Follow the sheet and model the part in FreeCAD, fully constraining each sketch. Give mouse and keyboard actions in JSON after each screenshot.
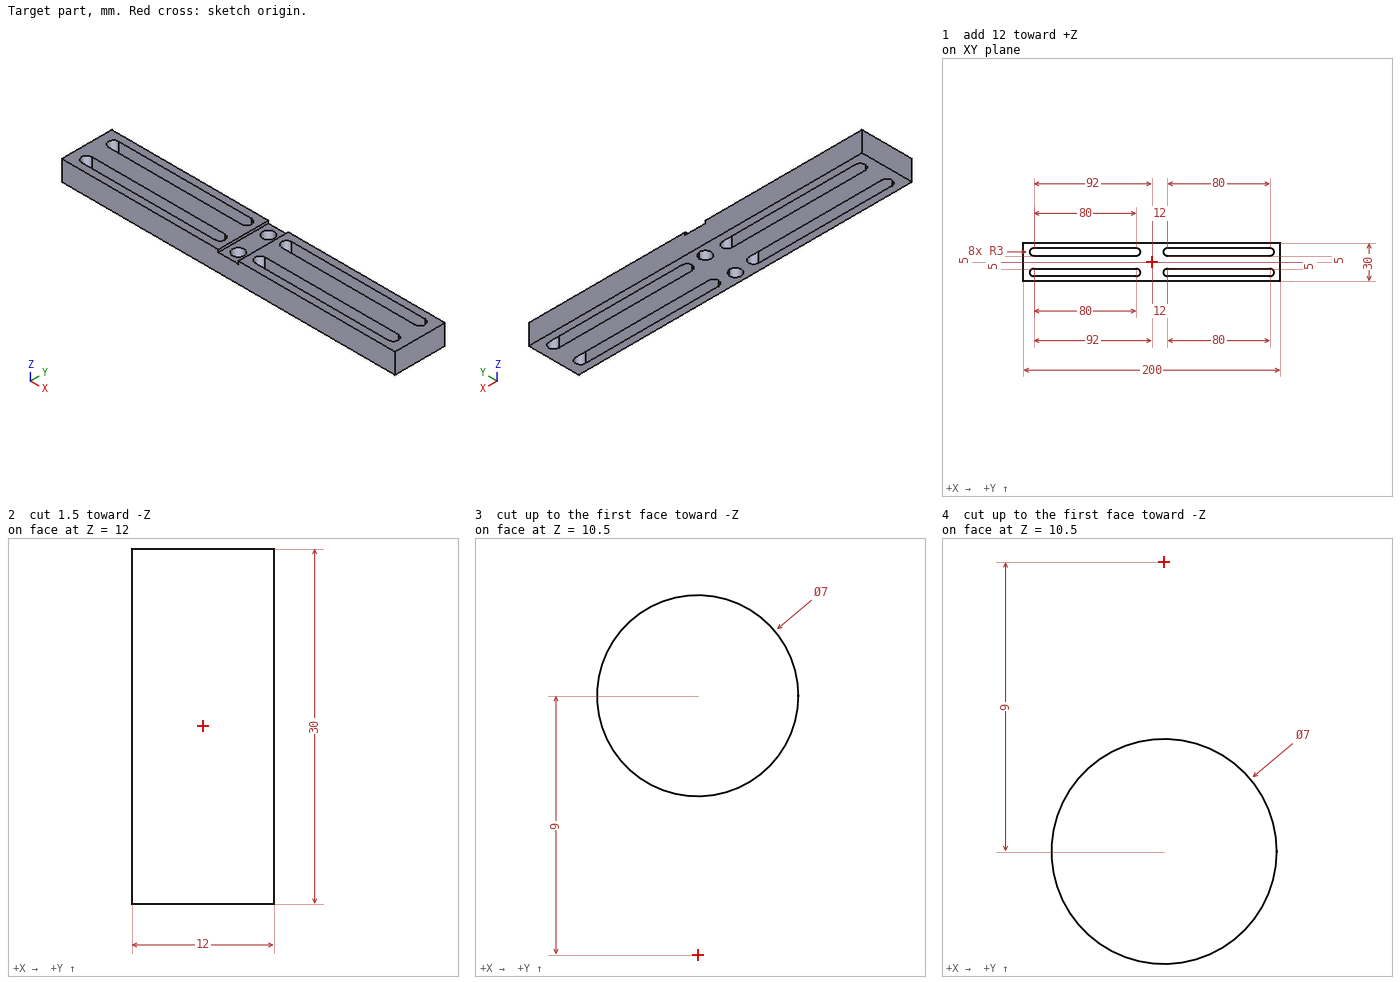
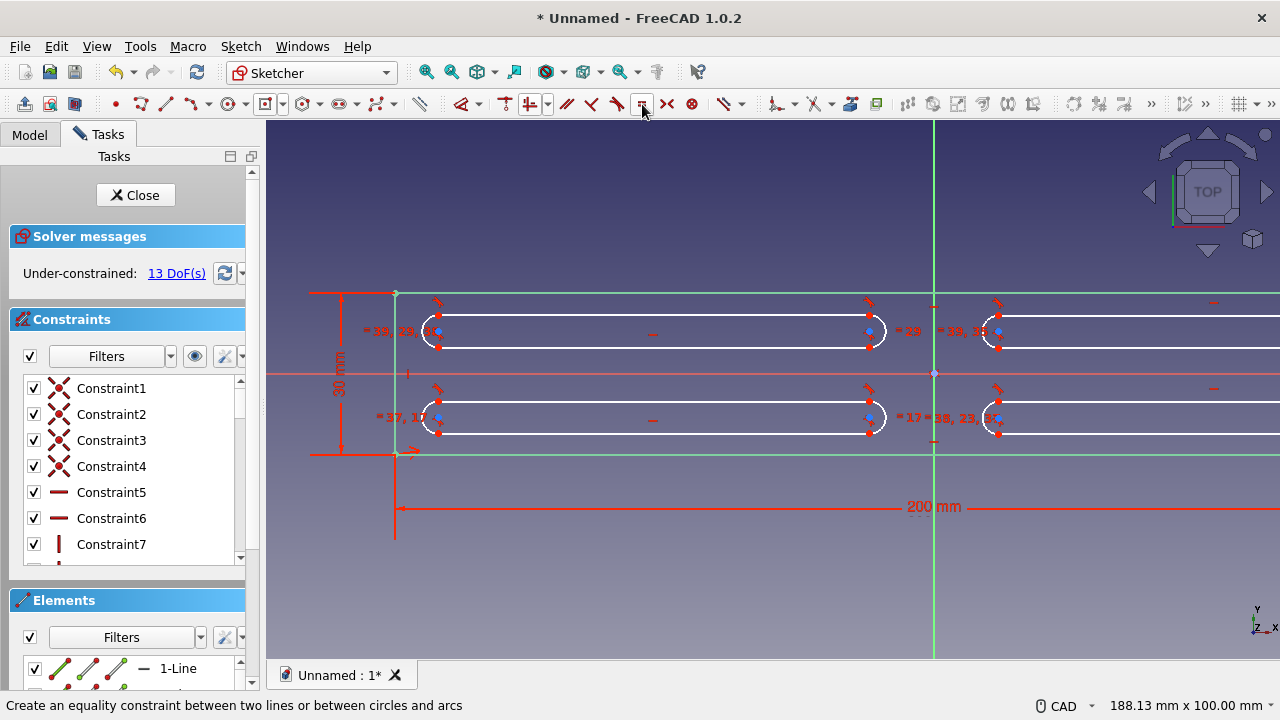
{"action": "left_click", "coordinate": [460, 104]}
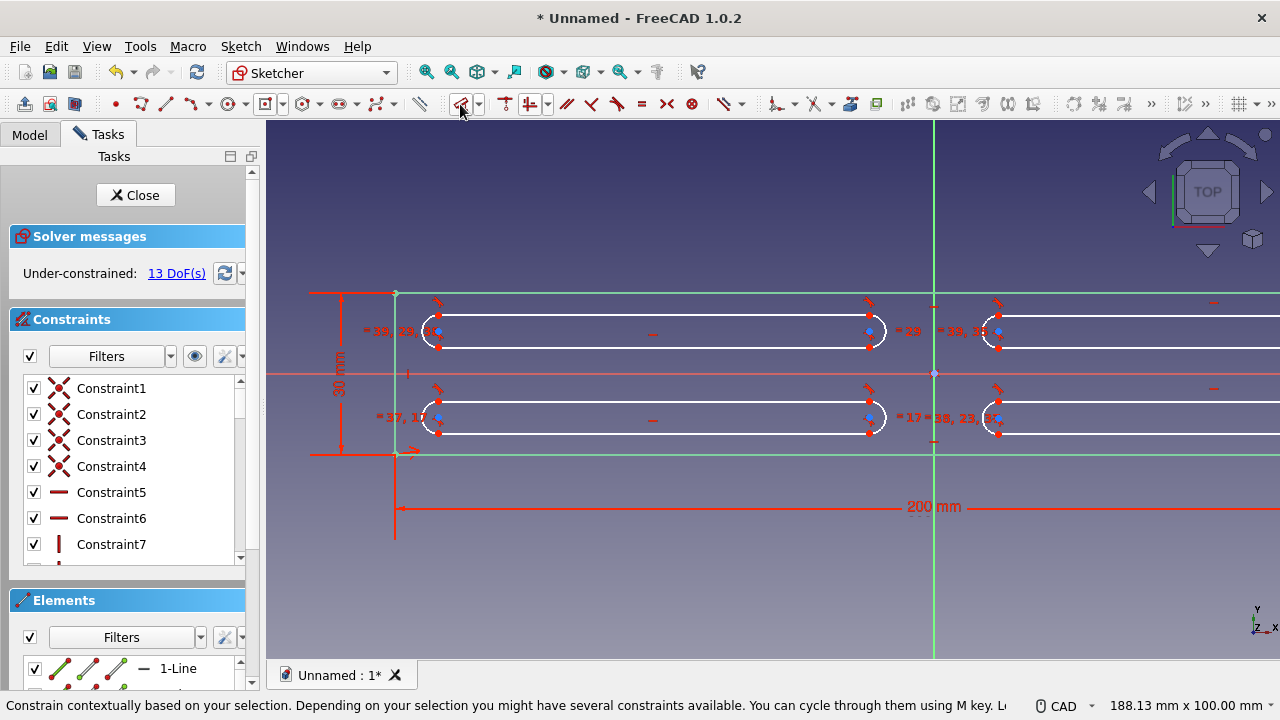
{"action": "scroll", "coordinate": [425, 408], "scroll_direction": "up", "scroll_amount": 5}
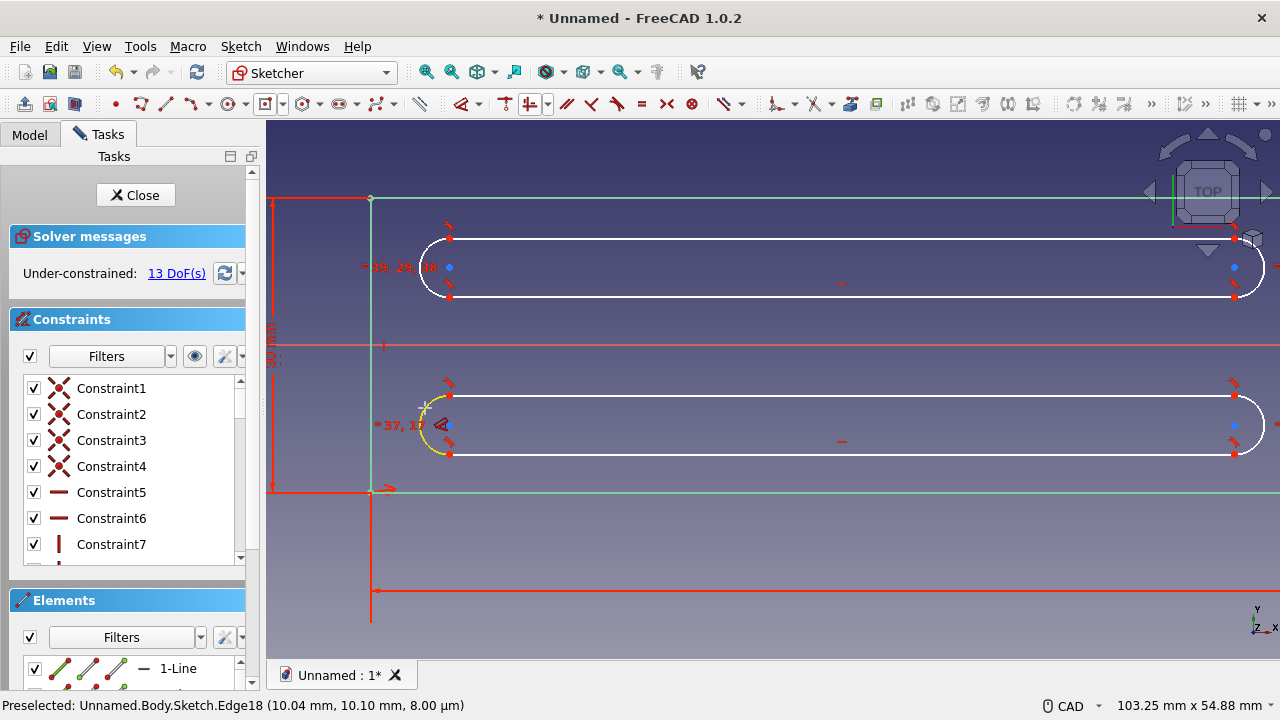
{"action": "left_click", "coordinate": [426, 408]}
{"action": "left_click", "coordinate": [400, 389]}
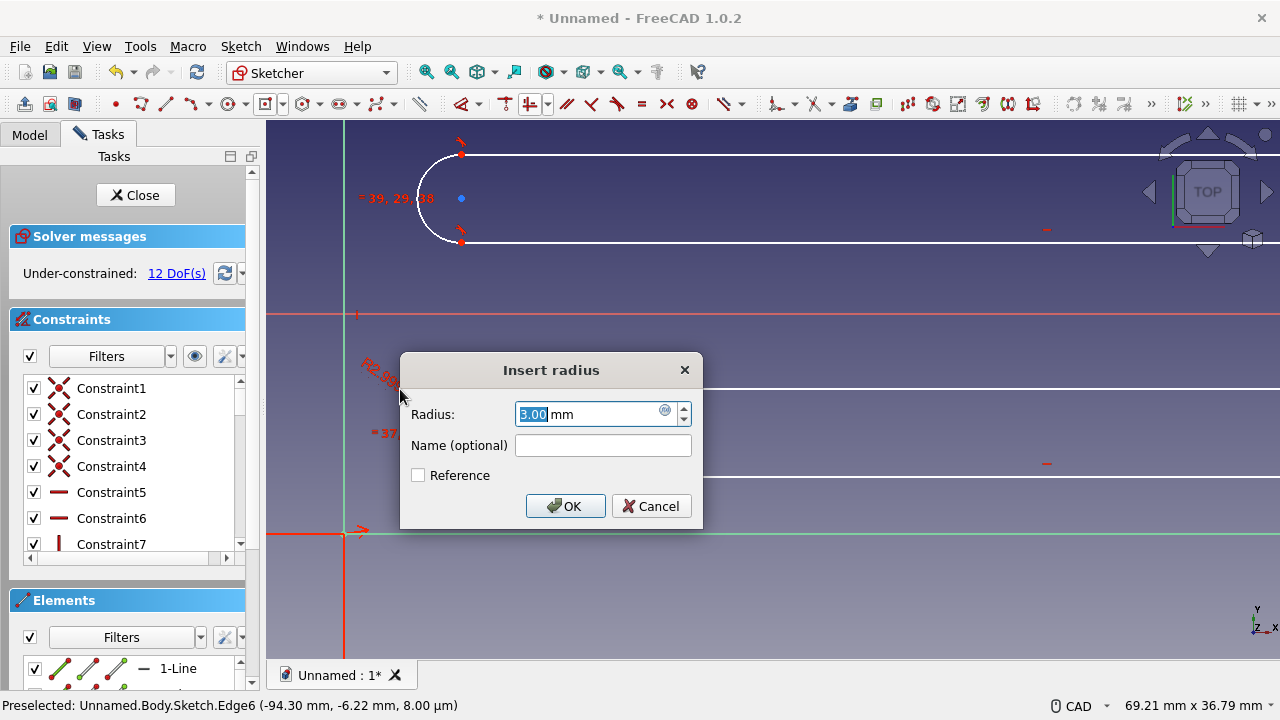
{"action": "type", "text": "3"}
{"action": "key", "text": "Return"}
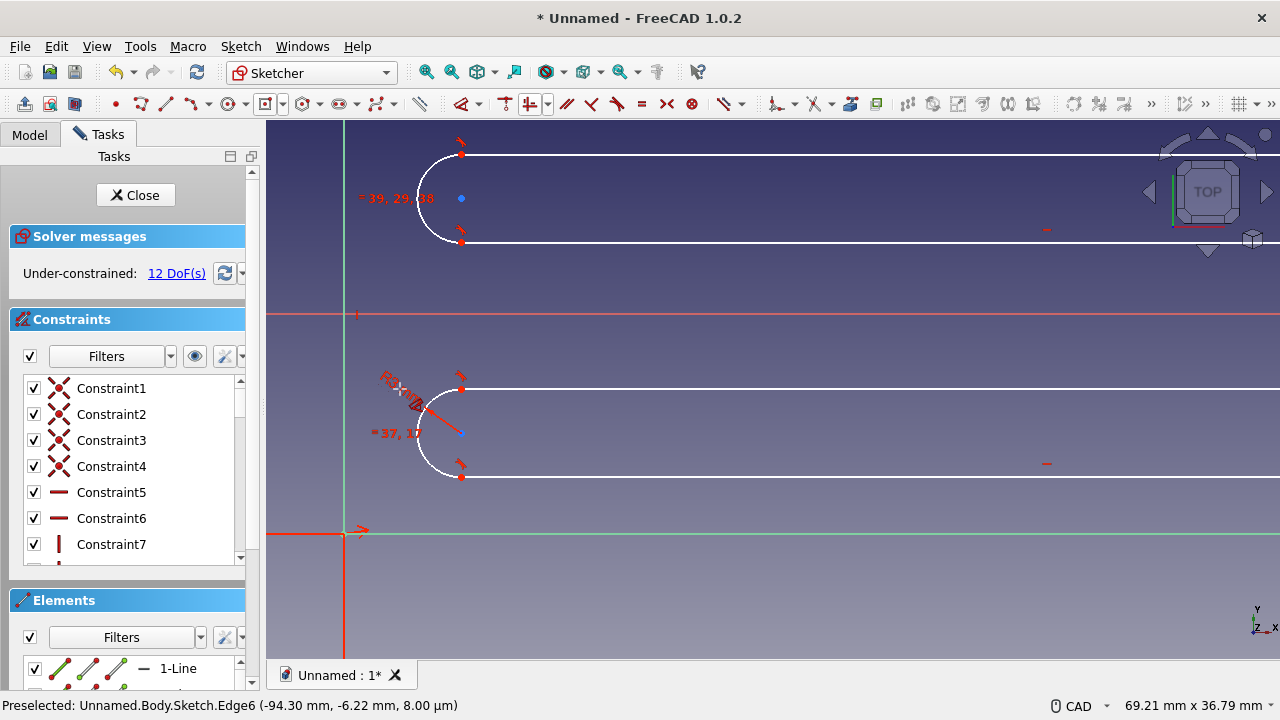
{"action": "scroll", "coordinate": [425, 409], "scroll_direction": "down", "scroll_amount": 8}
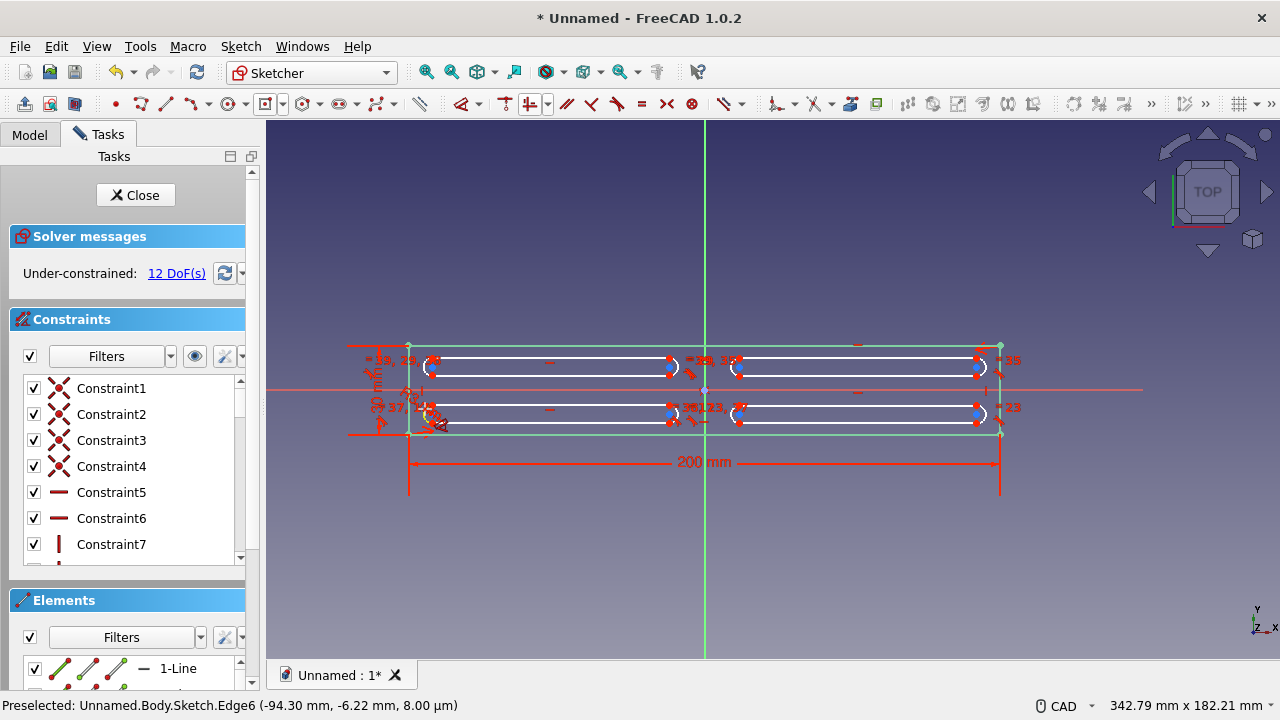
{"action": "left_click", "coordinate": [503, 405]}
{"action": "left_click", "coordinate": [551, 463]}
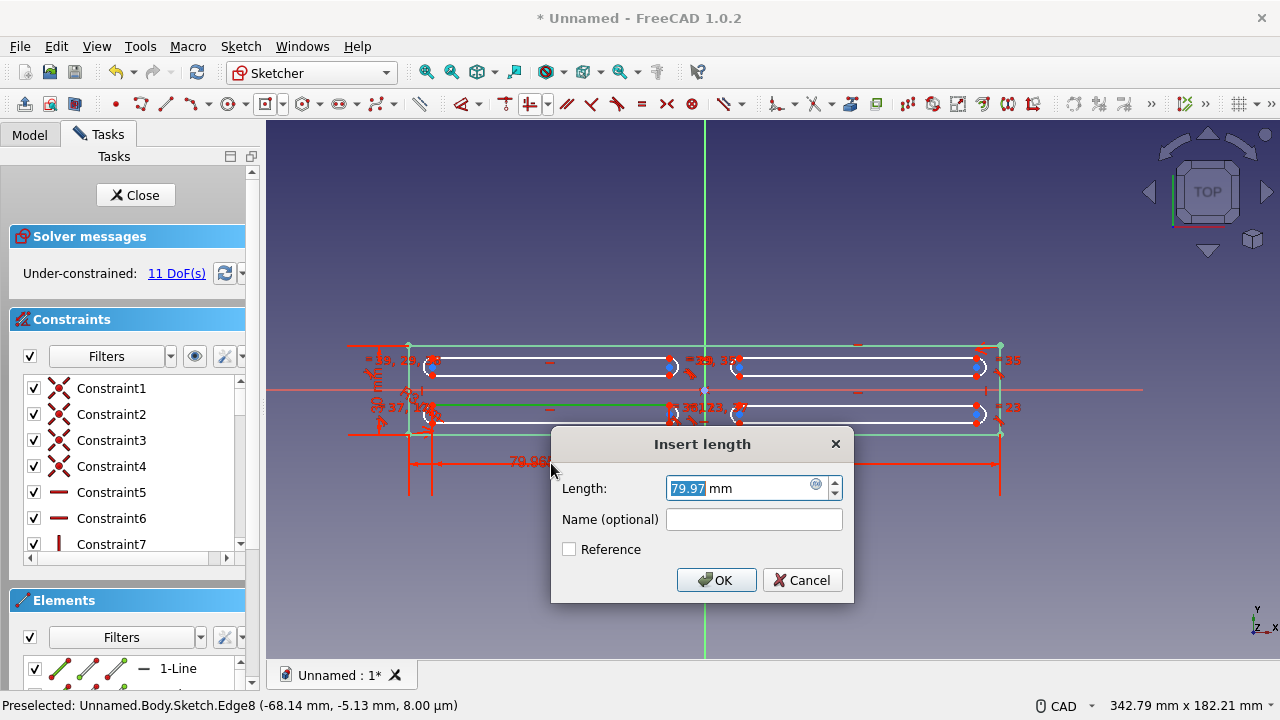
{"action": "type", "text": "80"}
{"action": "key", "text": "Return"}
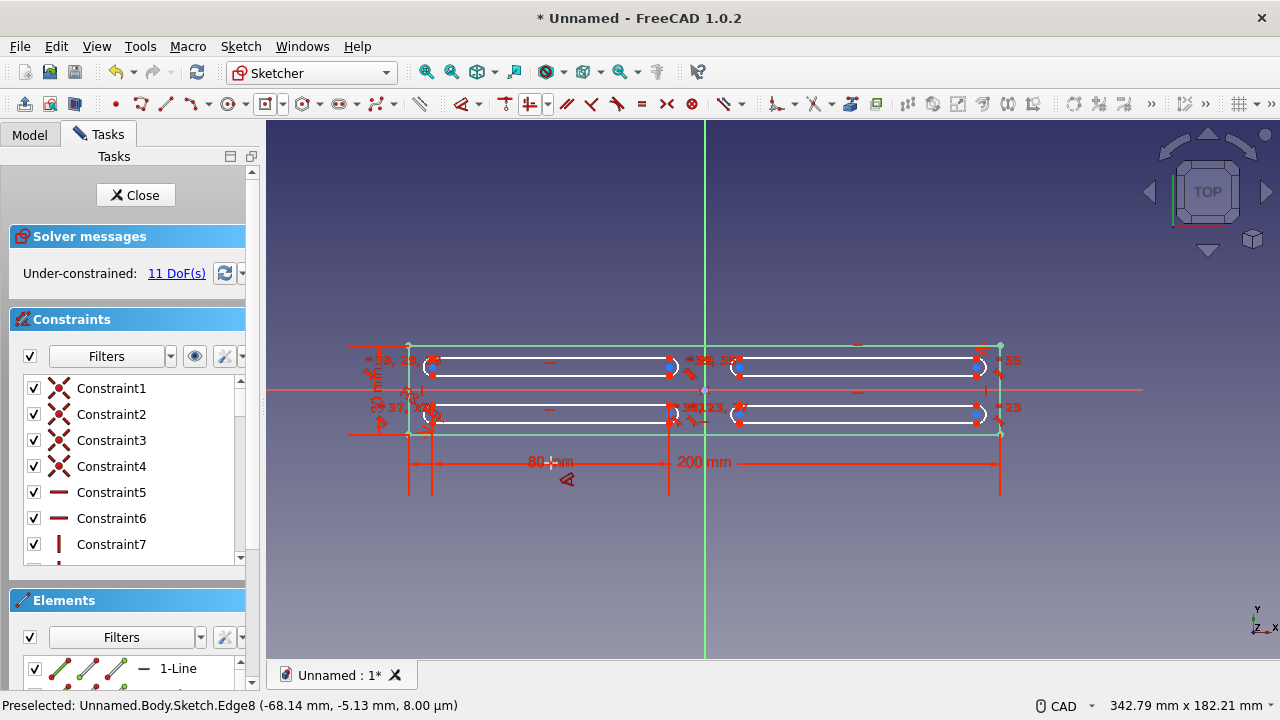
{"action": "left_click", "coordinate": [811, 406]}
{"action": "left_click", "coordinate": [858, 464]}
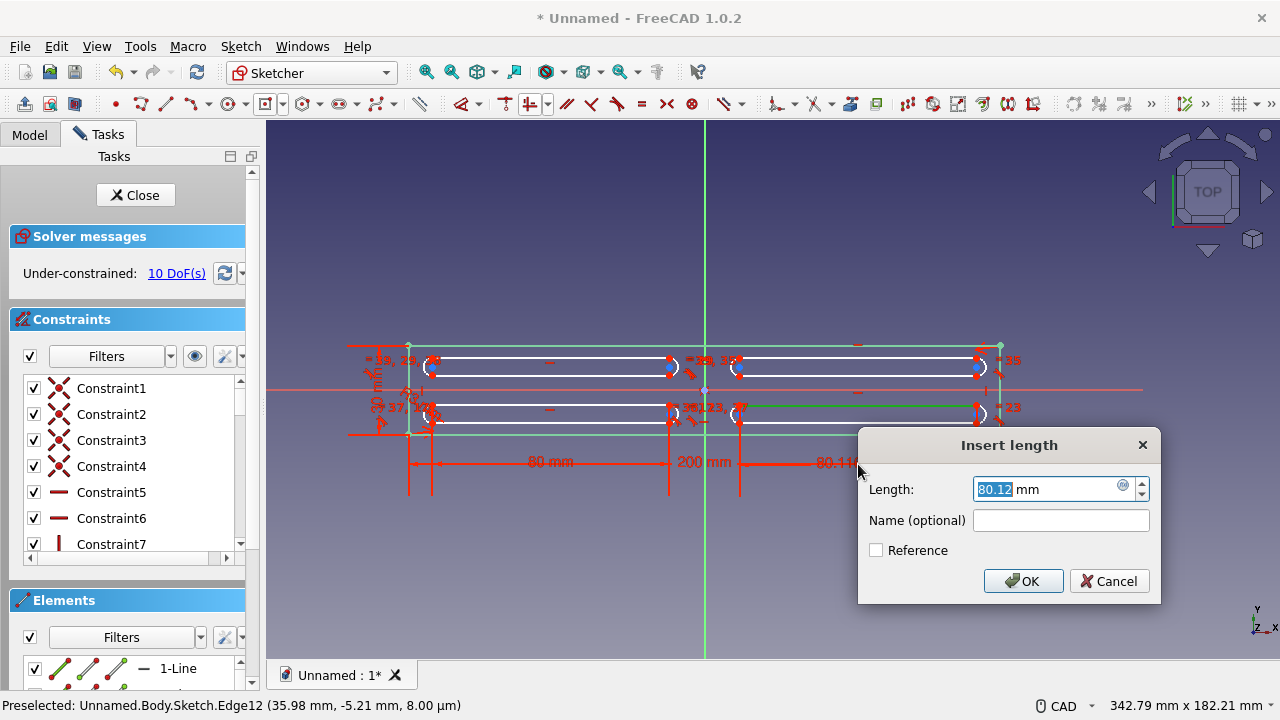
{"action": "type", "text": "80"}
{"action": "key", "text": "Return"}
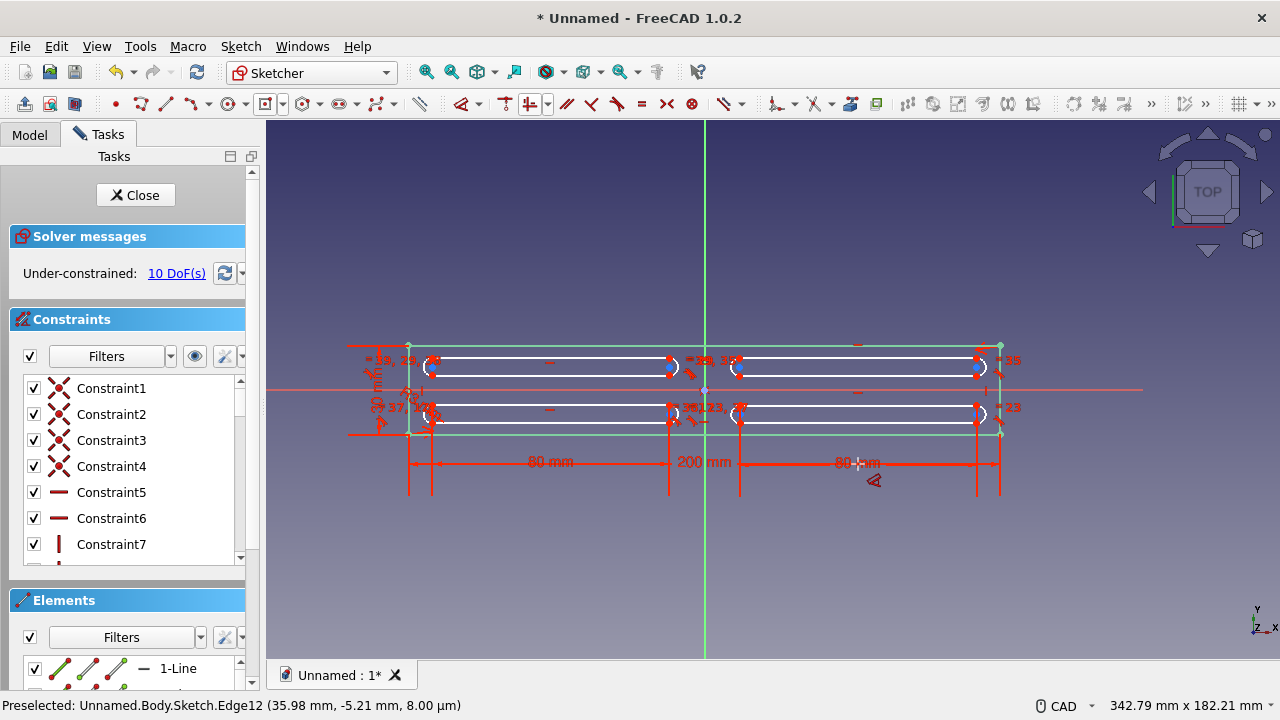
{"action": "left_click", "coordinate": [503, 358]}
{"action": "left_click", "coordinate": [551, 324]}